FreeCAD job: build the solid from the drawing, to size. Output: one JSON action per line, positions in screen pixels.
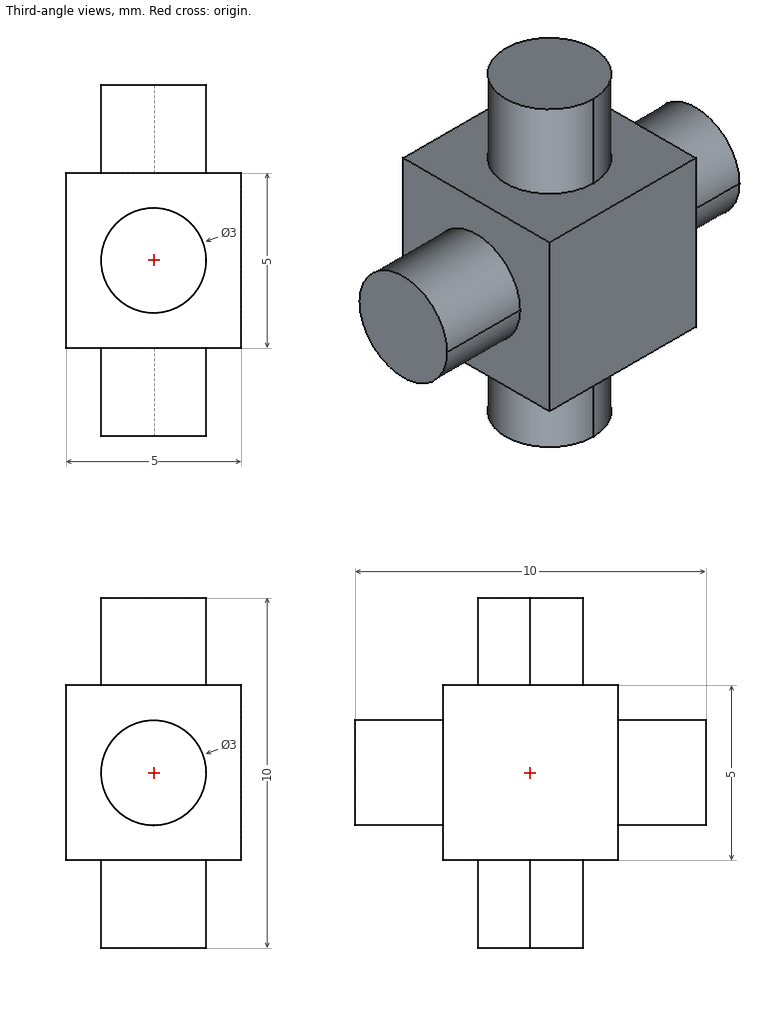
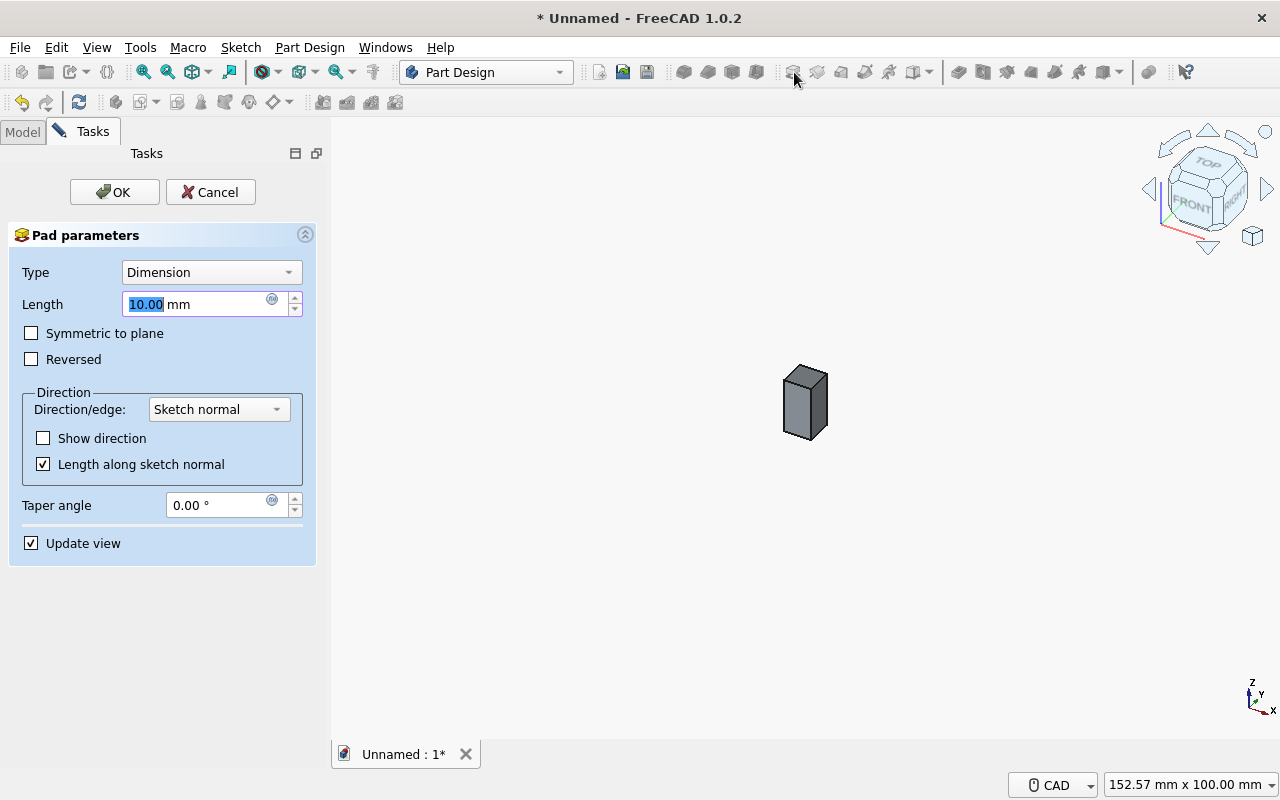
{"action": "type", "text": "5"}
{"action": "key", "text": "Tab"}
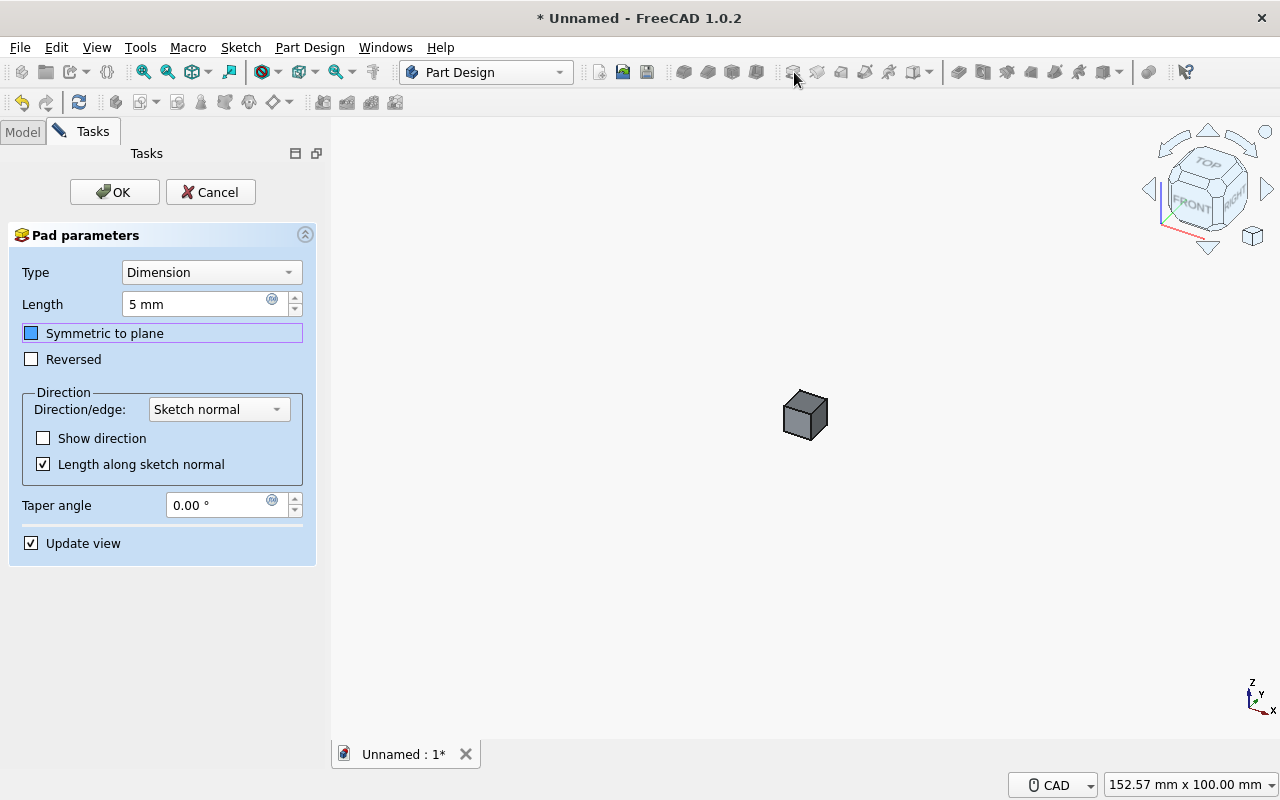
{"action": "left_click", "coordinate": [30, 333]}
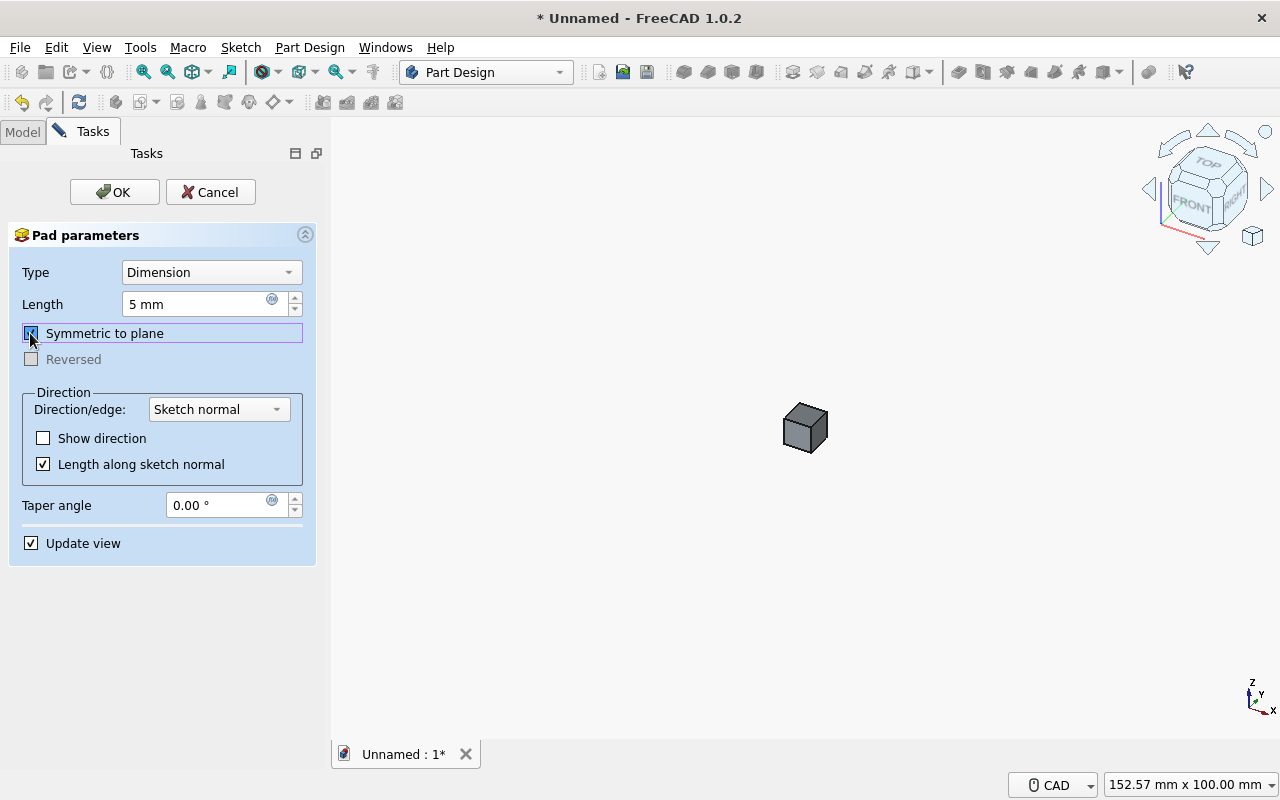
{"action": "left_click", "coordinate": [115, 192]}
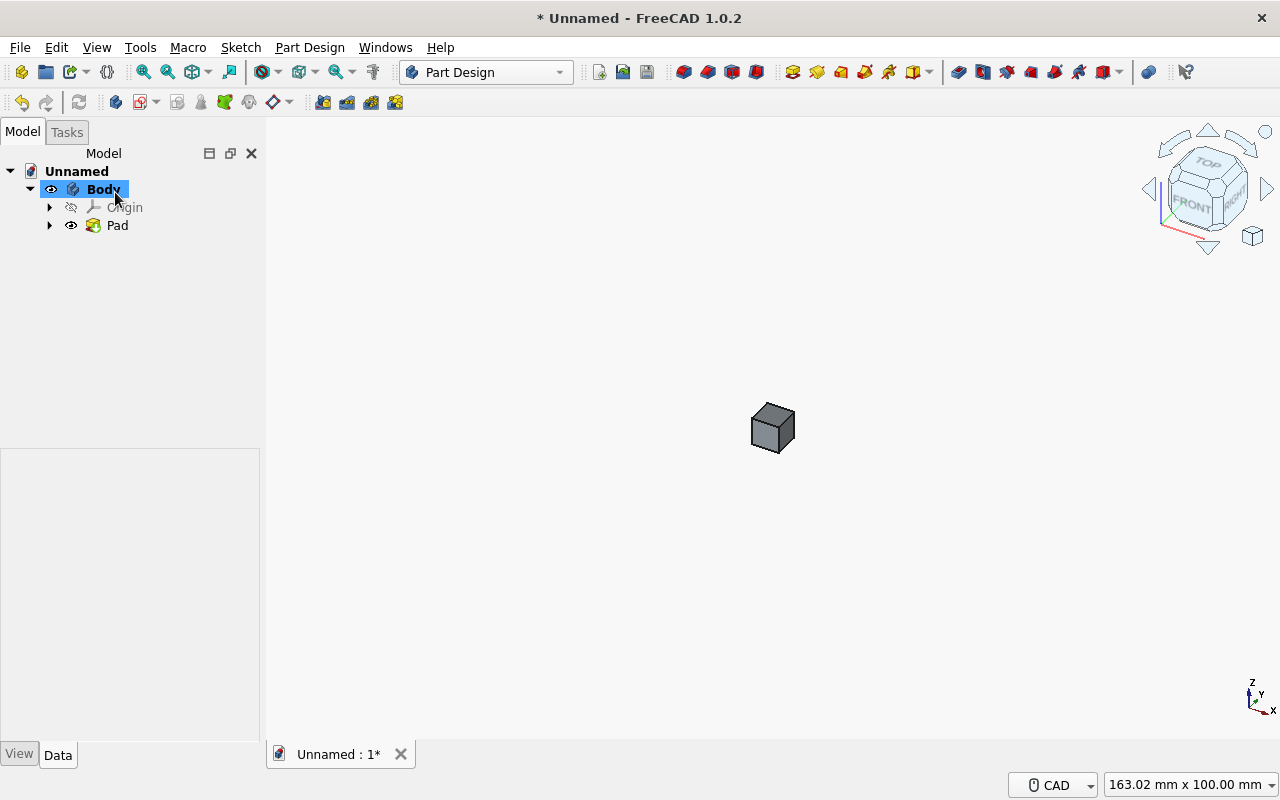
{"action": "left_click", "coordinate": [144, 72]}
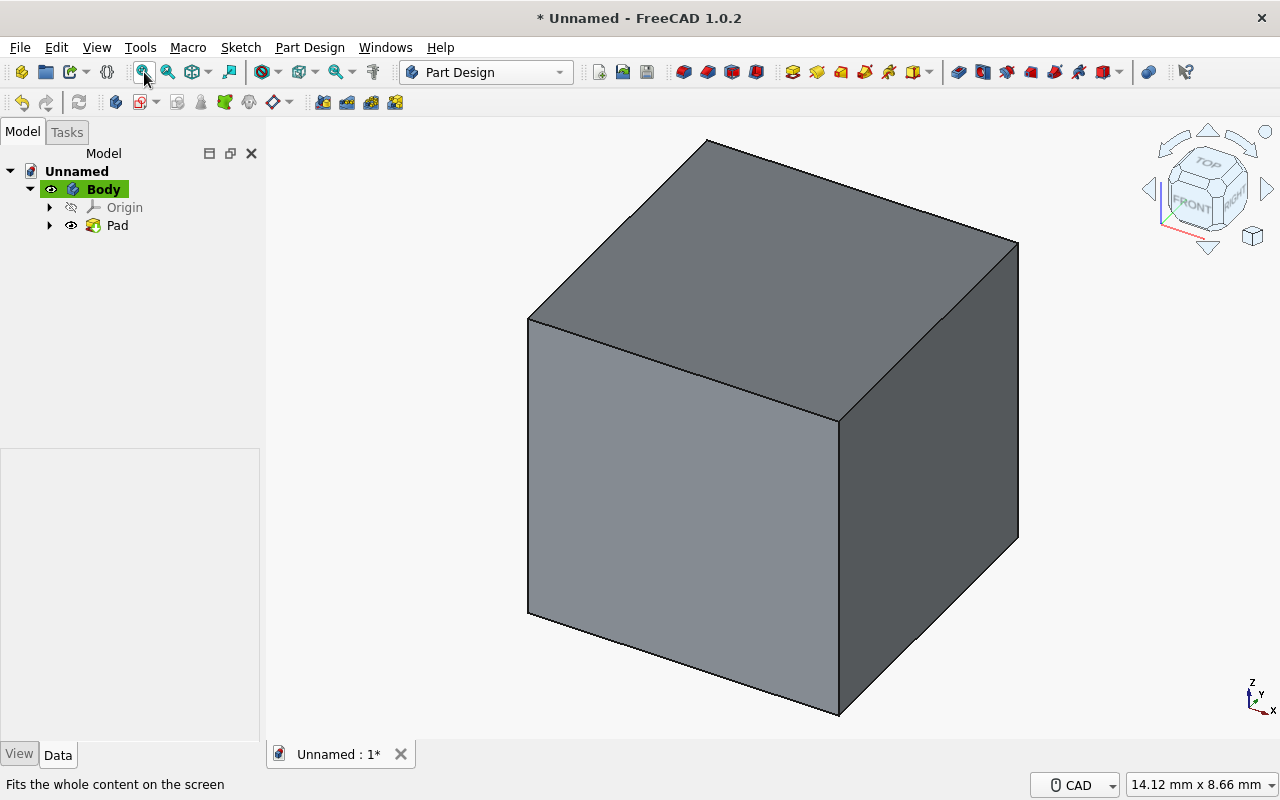
{"action": "left_click", "coordinate": [140, 102]}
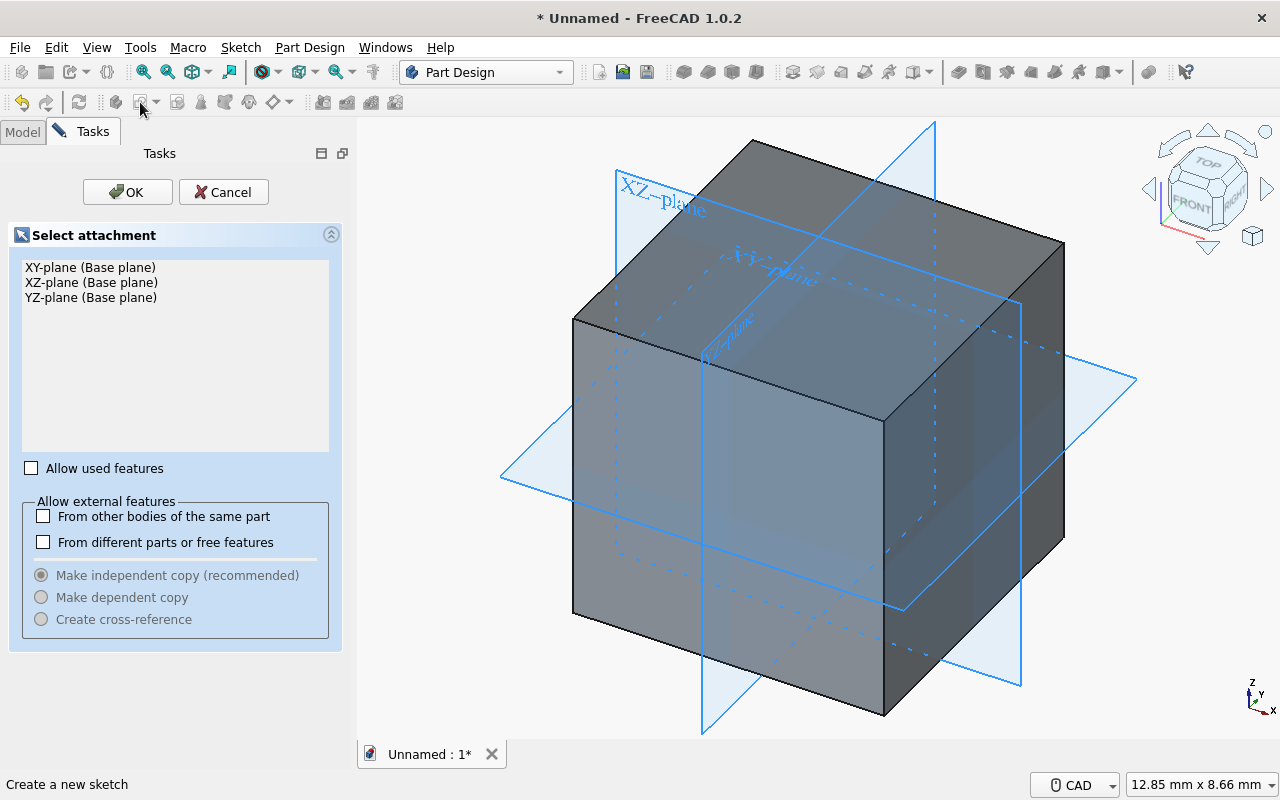
{"action": "left_click", "coordinate": [82, 282]}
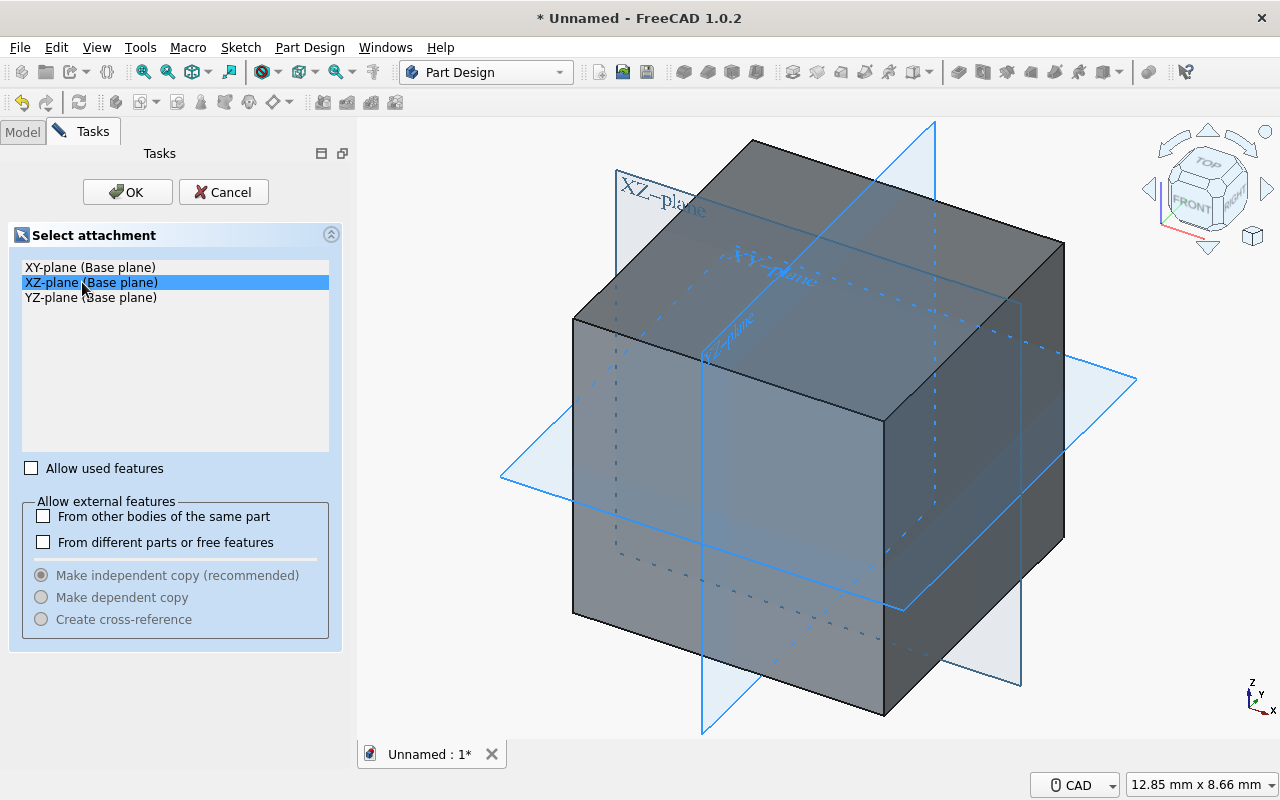
{"action": "left_click", "coordinate": [128, 192]}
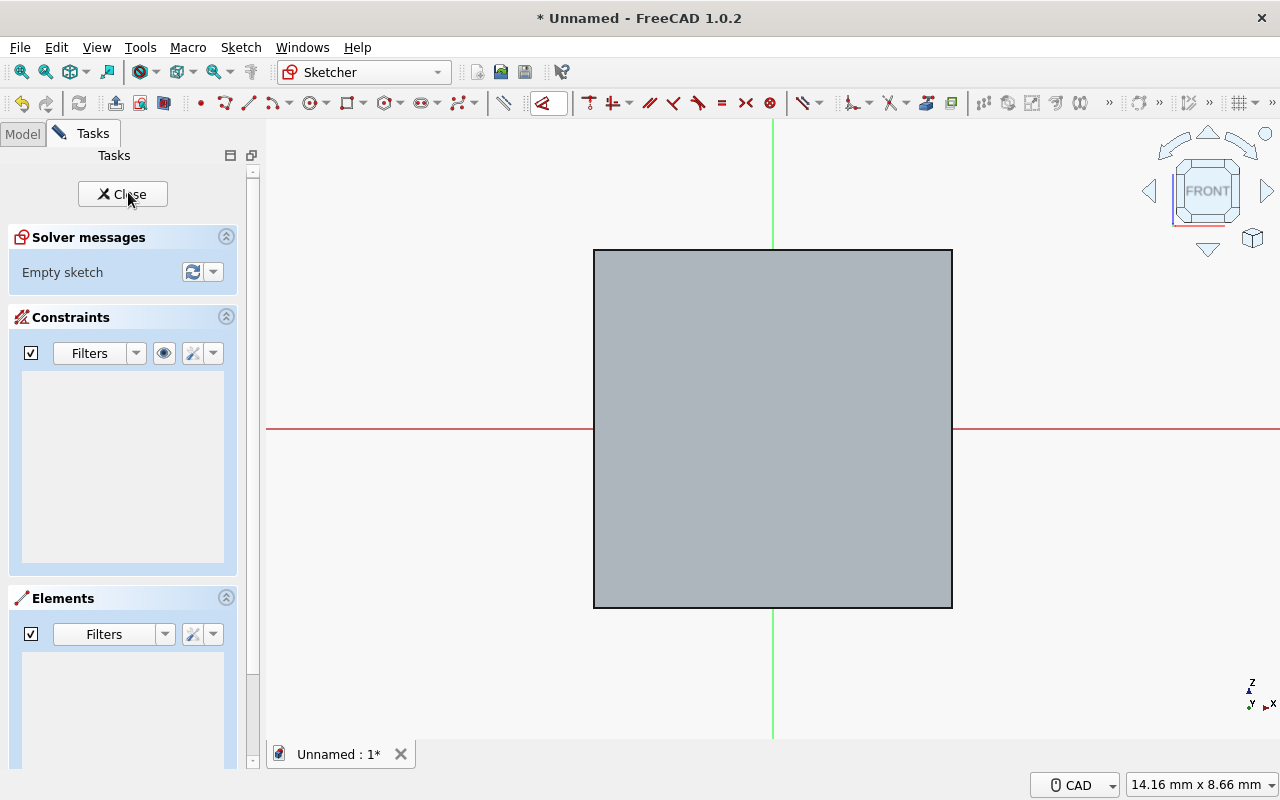
{"action": "left_click", "coordinate": [164, 104]}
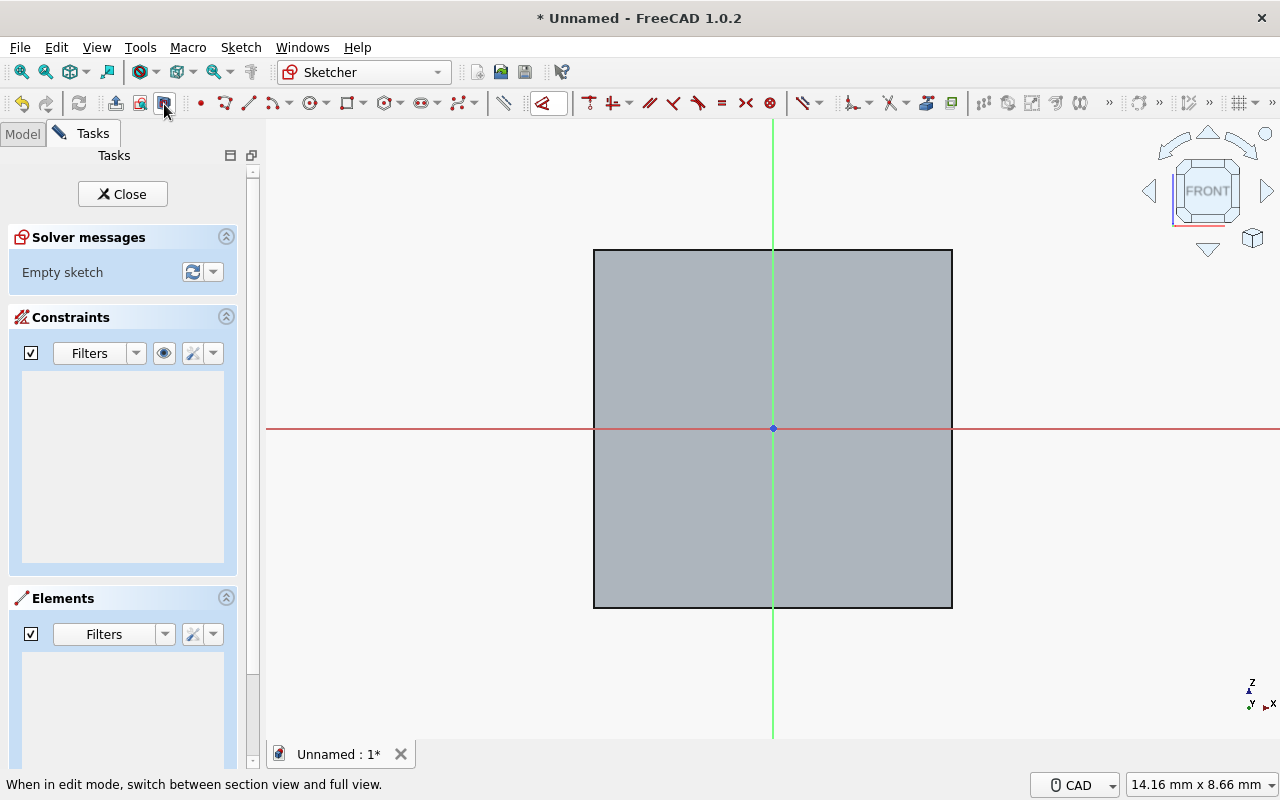
{"action": "scroll", "coordinate": [856, 429], "scroll_direction": "up", "scroll_amount": 3}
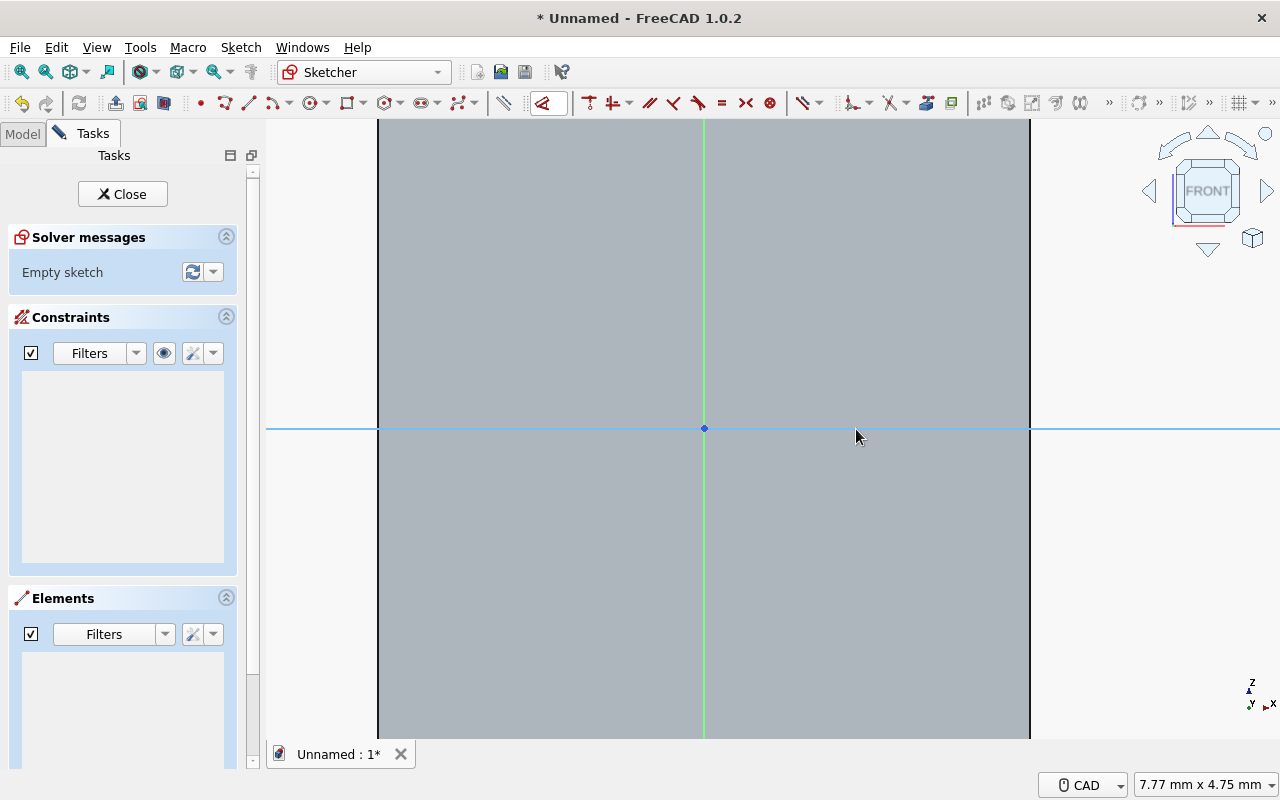
{"action": "left_click", "coordinate": [310, 104]}